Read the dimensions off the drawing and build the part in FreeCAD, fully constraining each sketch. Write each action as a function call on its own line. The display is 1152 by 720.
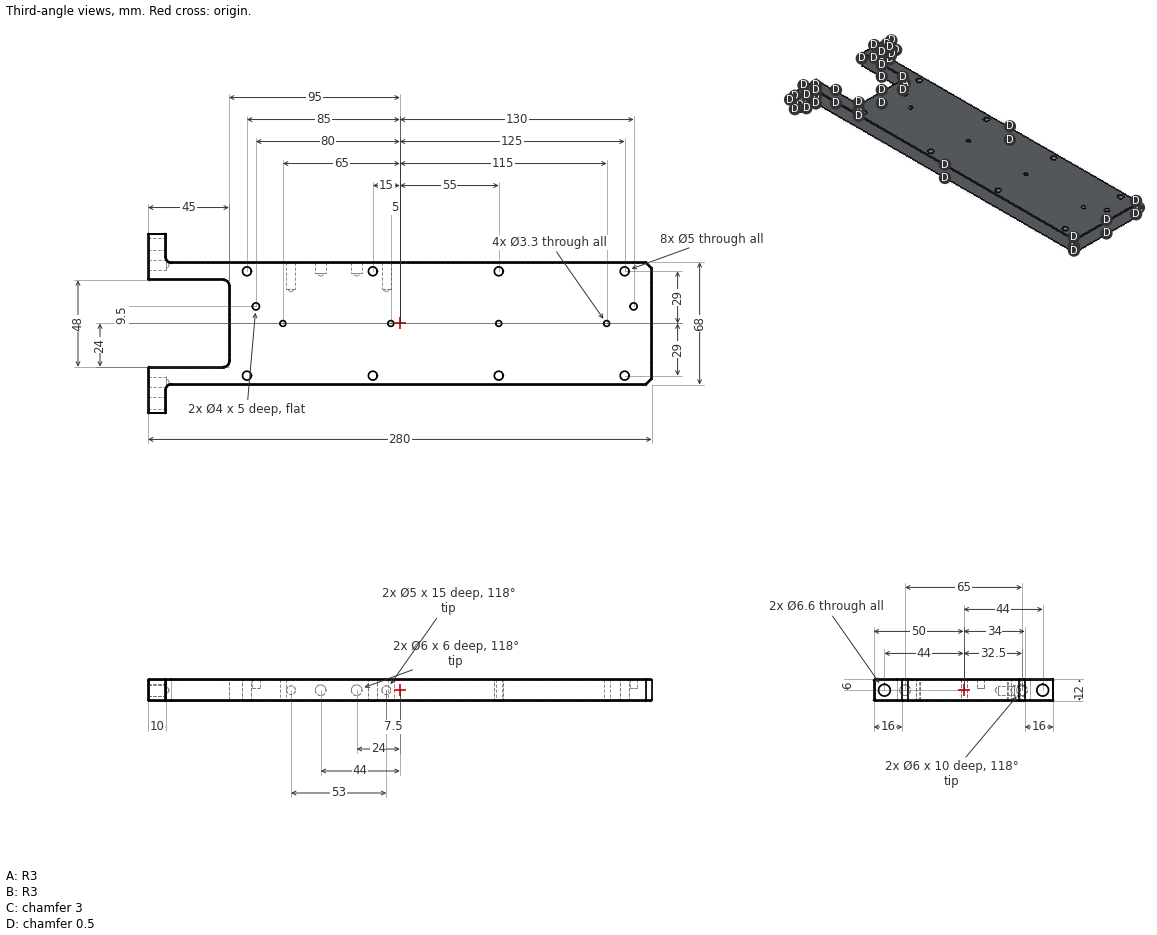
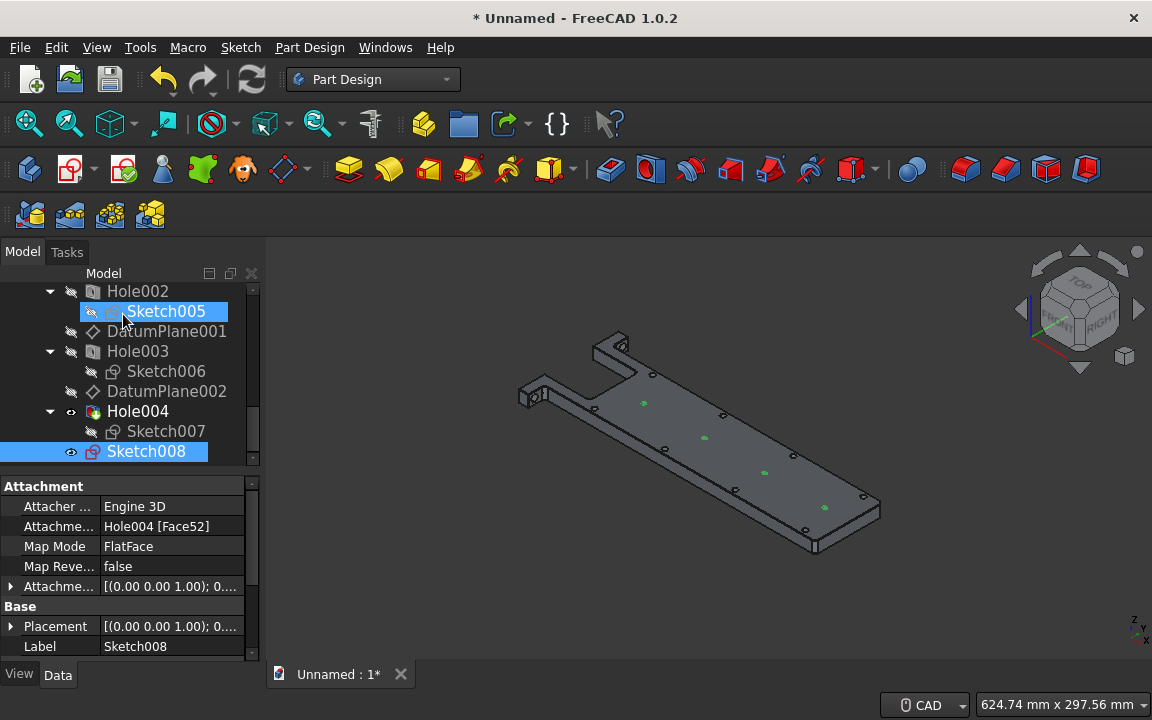
click(652, 170)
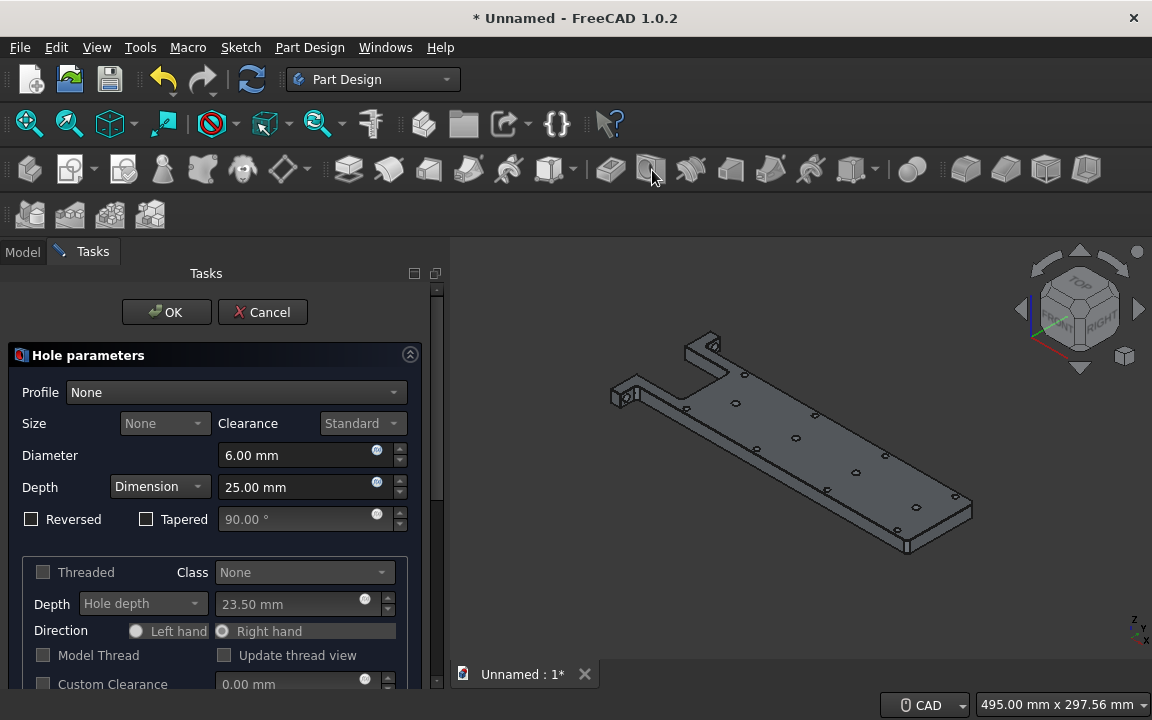
triple_click(305, 455)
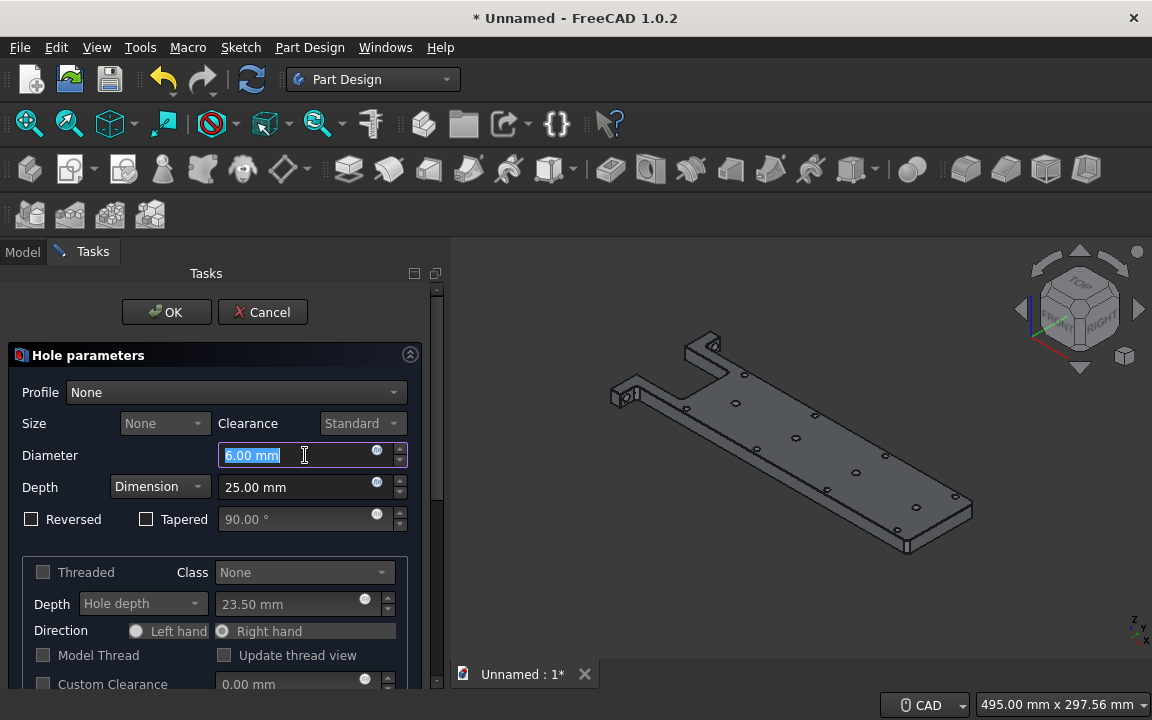
text(3.3)
key(Tab)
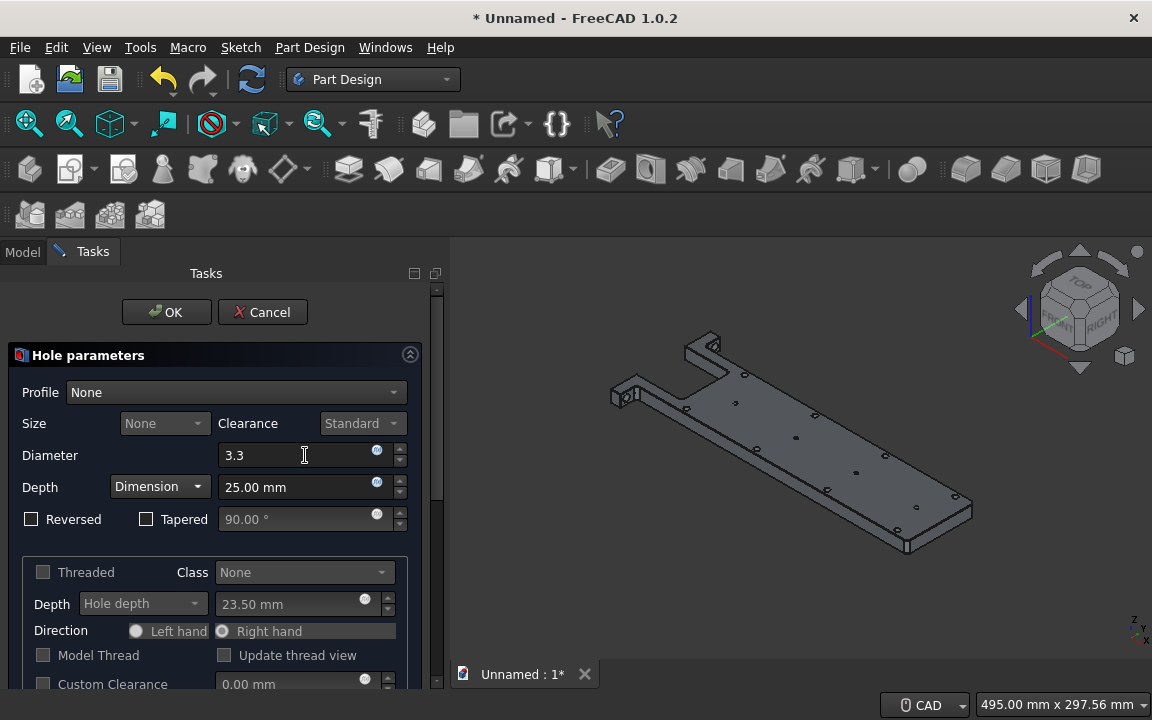
click(161, 486)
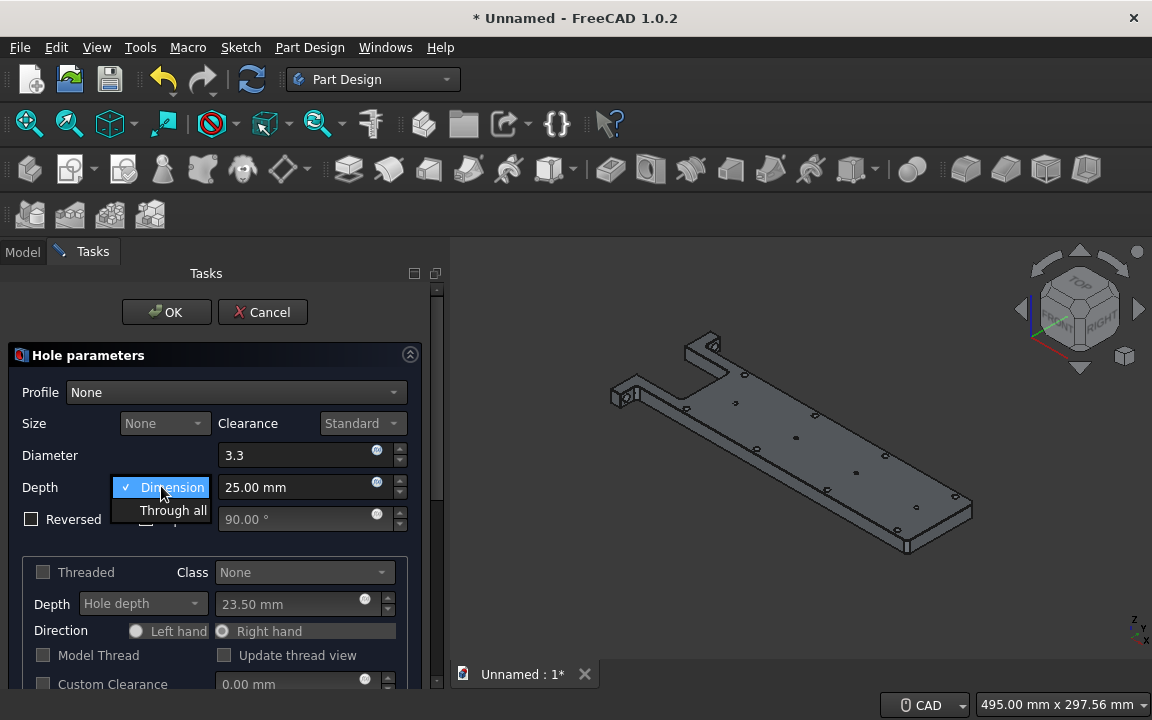
click(160, 510)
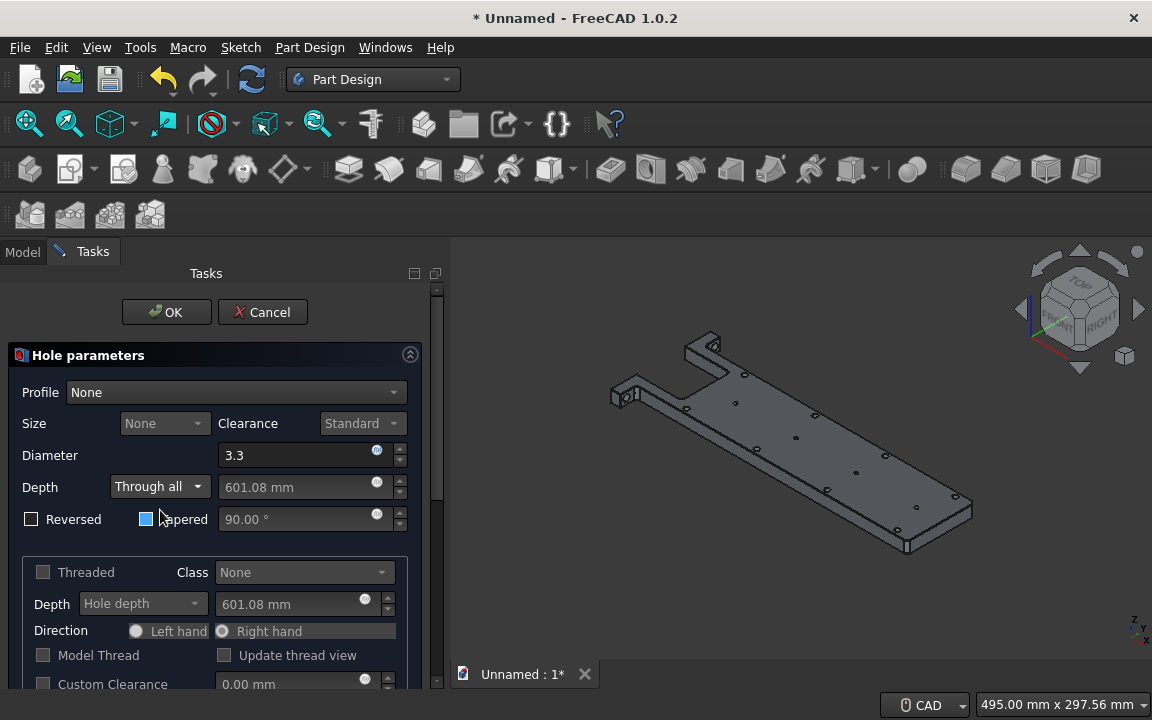
click(167, 312)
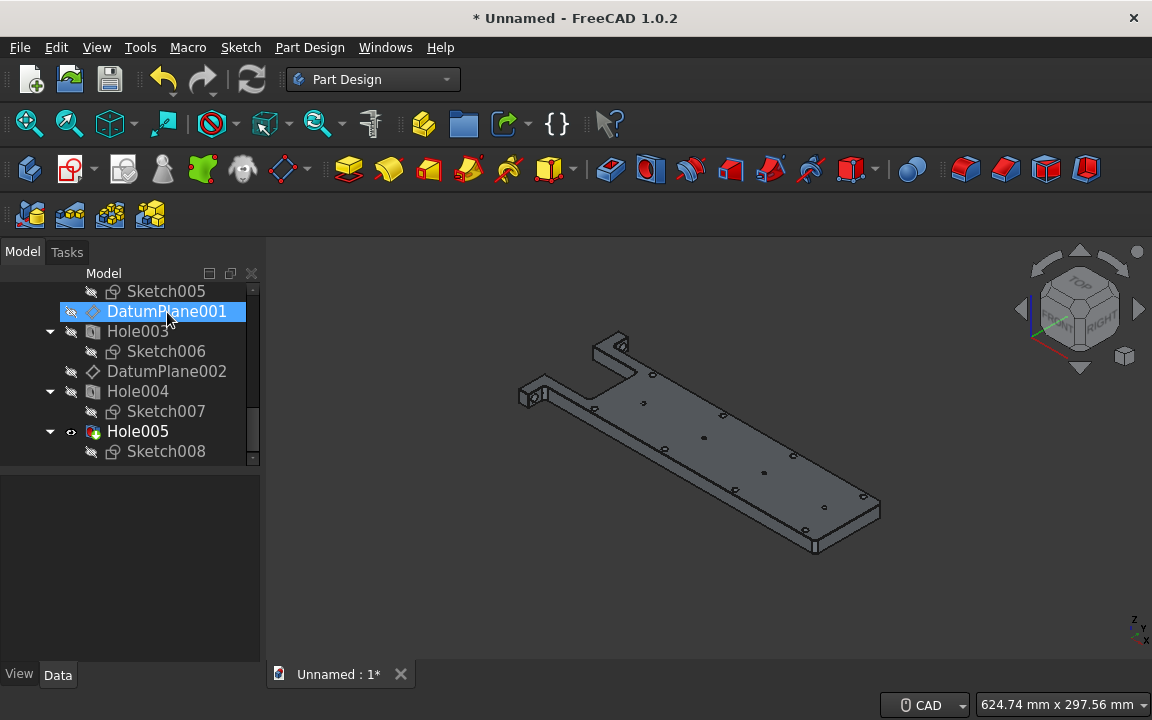
click(669, 417)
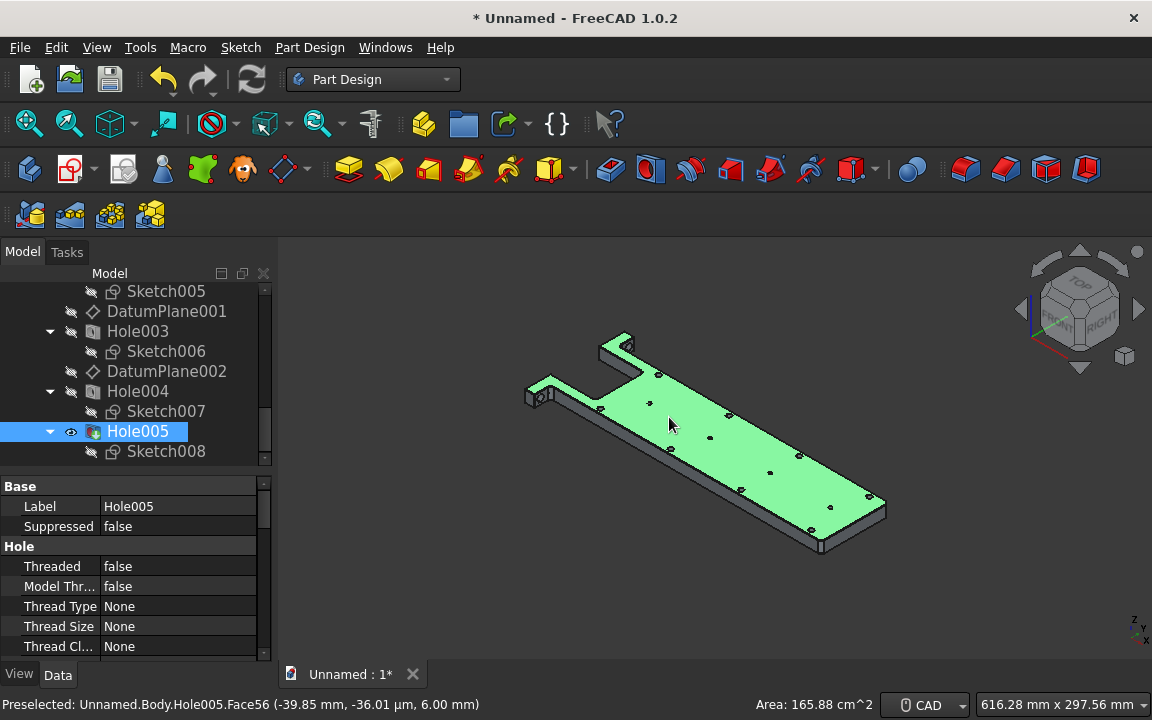
click(70, 170)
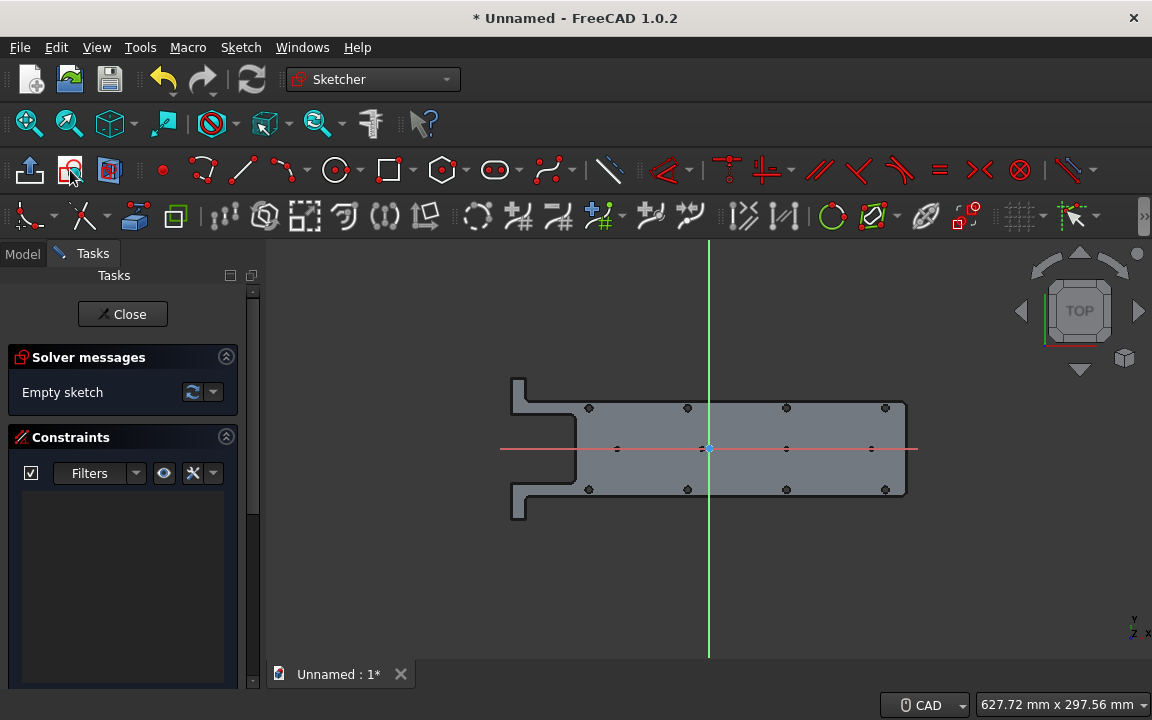
scroll(955, 424, up, 2)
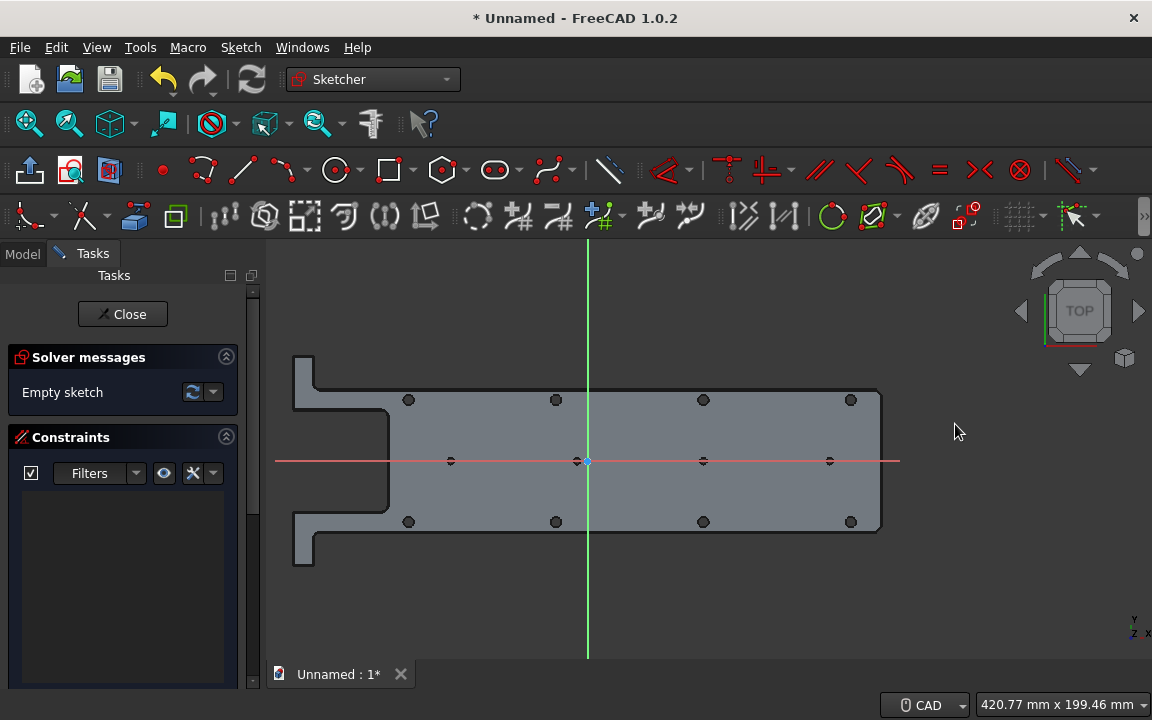
key(g)
key(c)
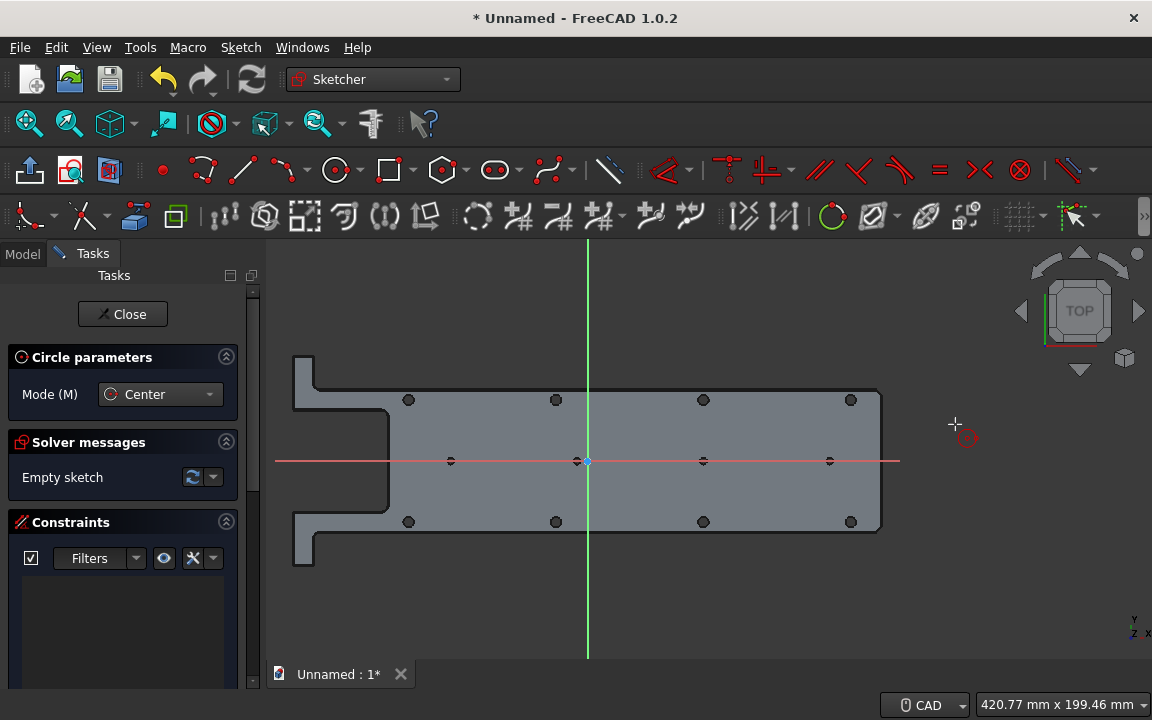
scroll(419, 441, up, 9)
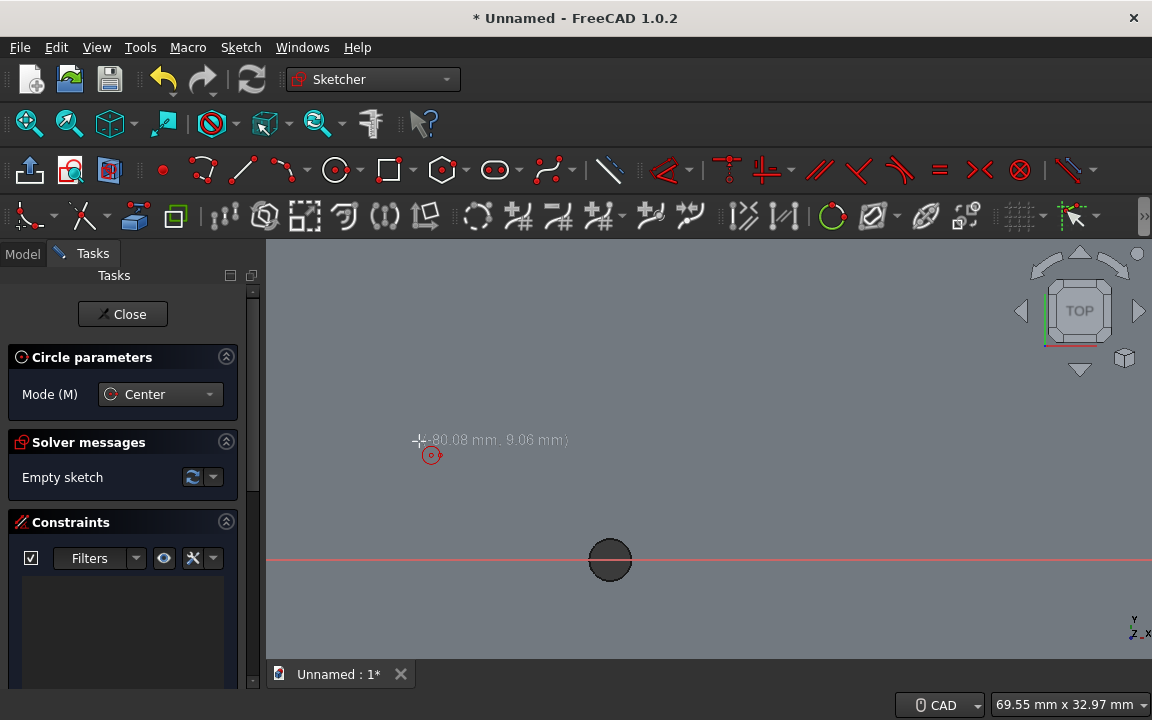
scroll(419, 442, down, 9)